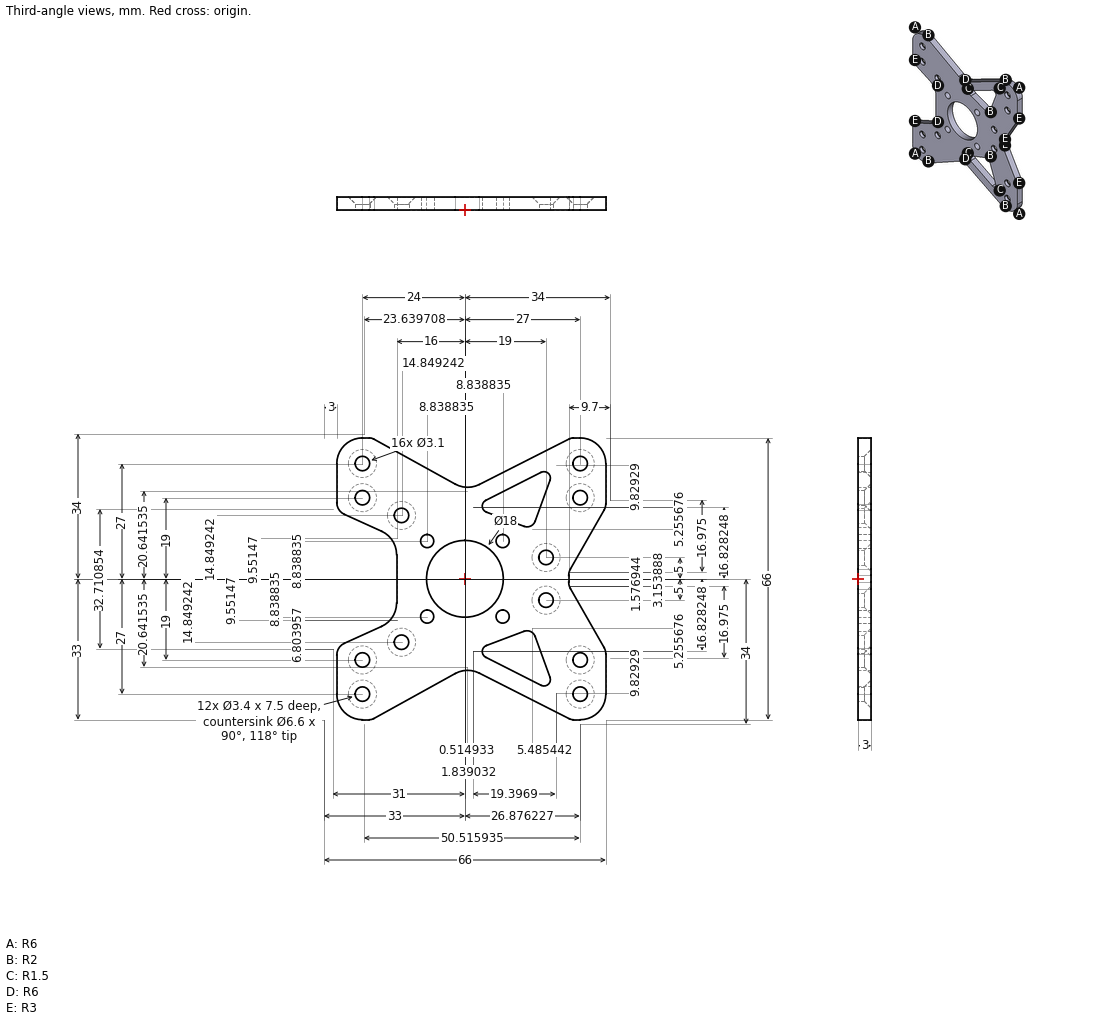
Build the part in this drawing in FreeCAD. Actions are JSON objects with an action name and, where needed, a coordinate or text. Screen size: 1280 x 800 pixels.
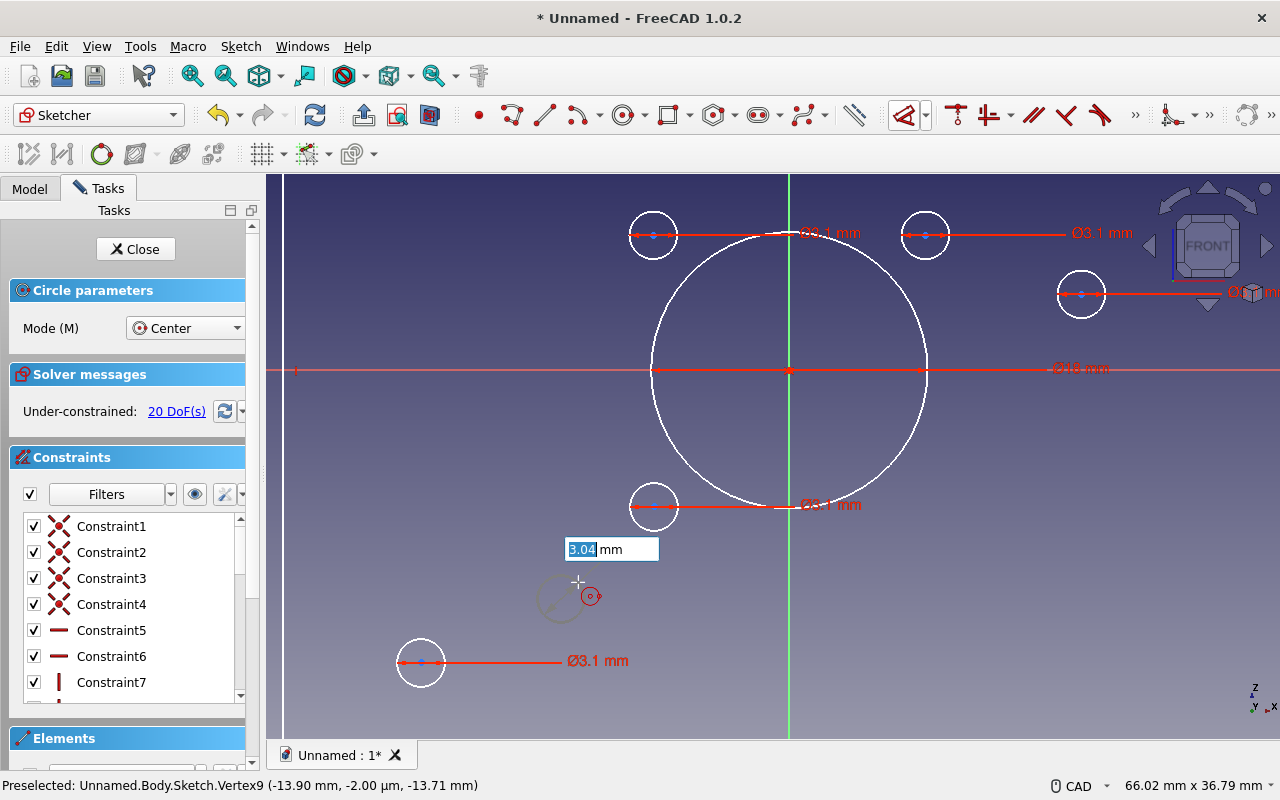
{"action": "type", "text": "3.1"}
{"action": "key", "text": "Return"}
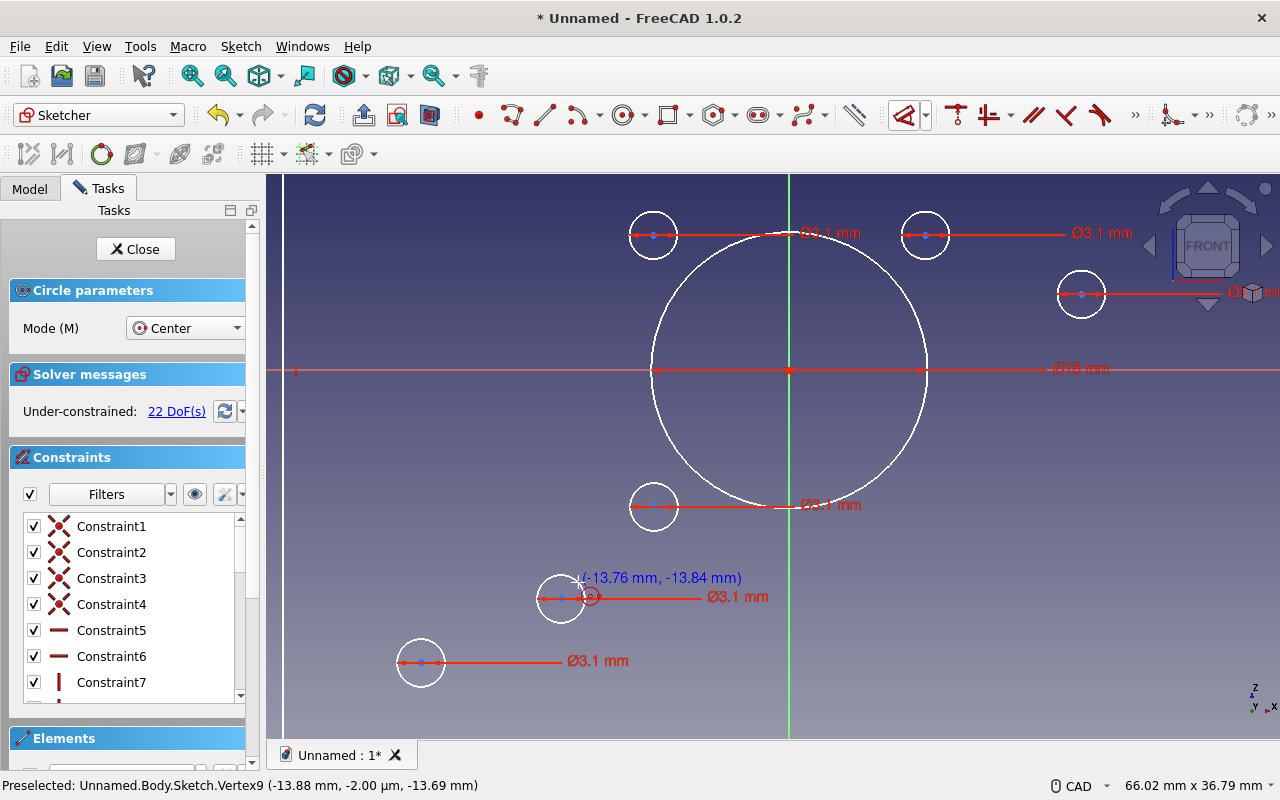
{"action": "scroll", "coordinate": [655, 507], "scroll_direction": "down", "scroll_amount": 5}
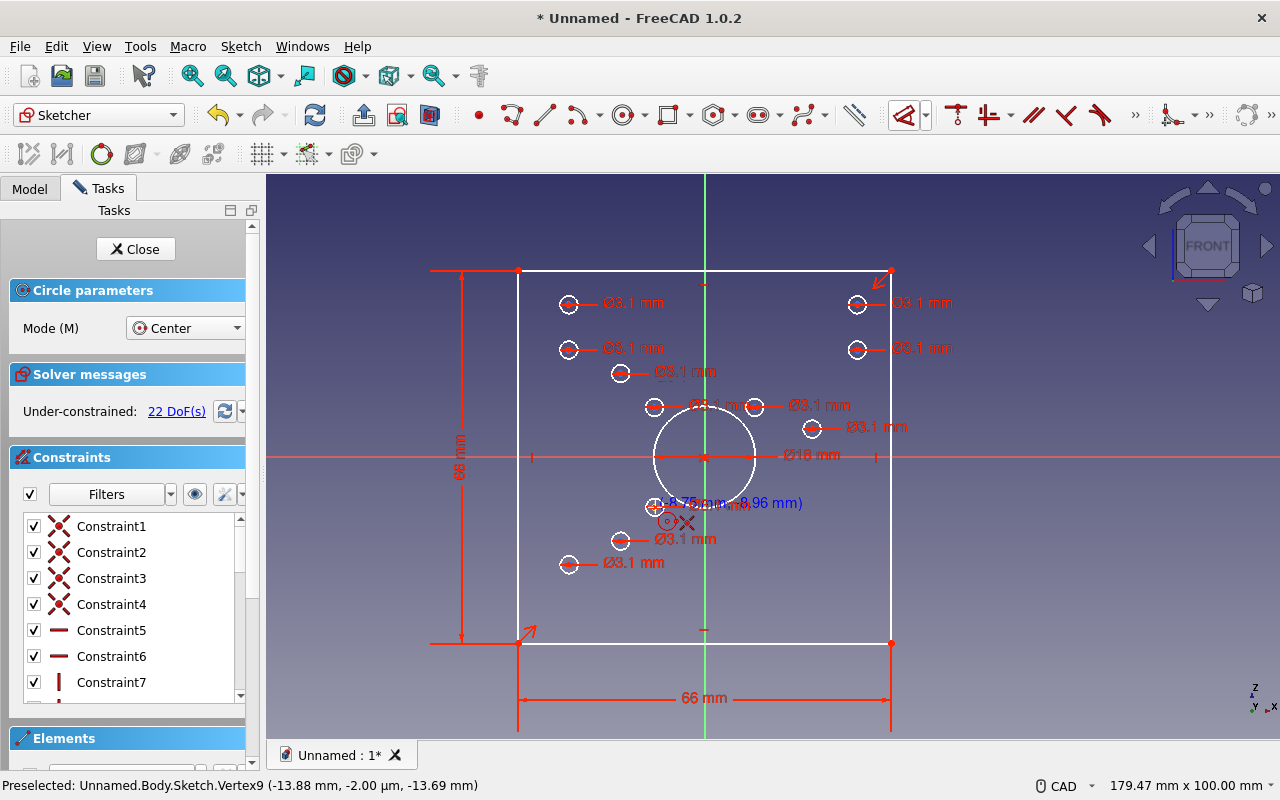
{"action": "scroll", "coordinate": [569, 610], "scroll_direction": "up", "scroll_amount": 5}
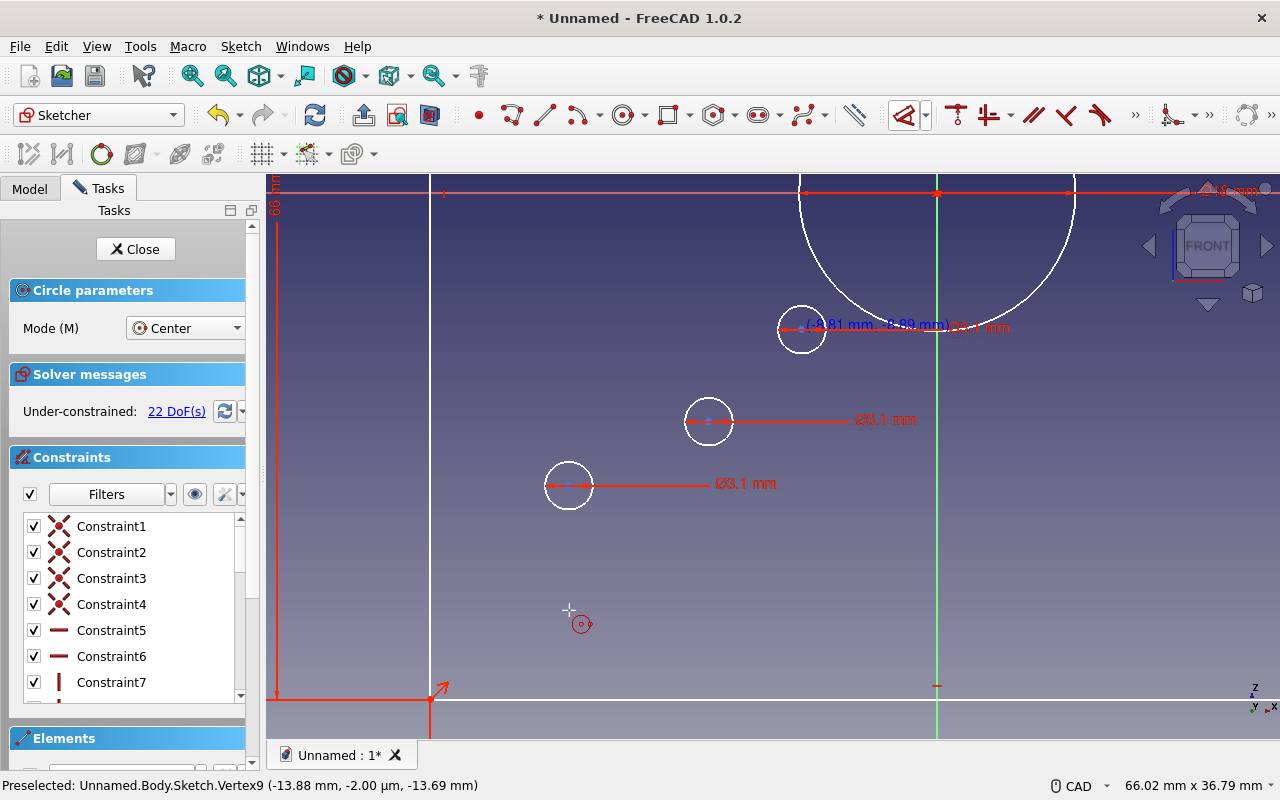
{"action": "left_click", "coordinate": [569, 608]}
{"action": "mouse_move", "coordinate": [585, 591]}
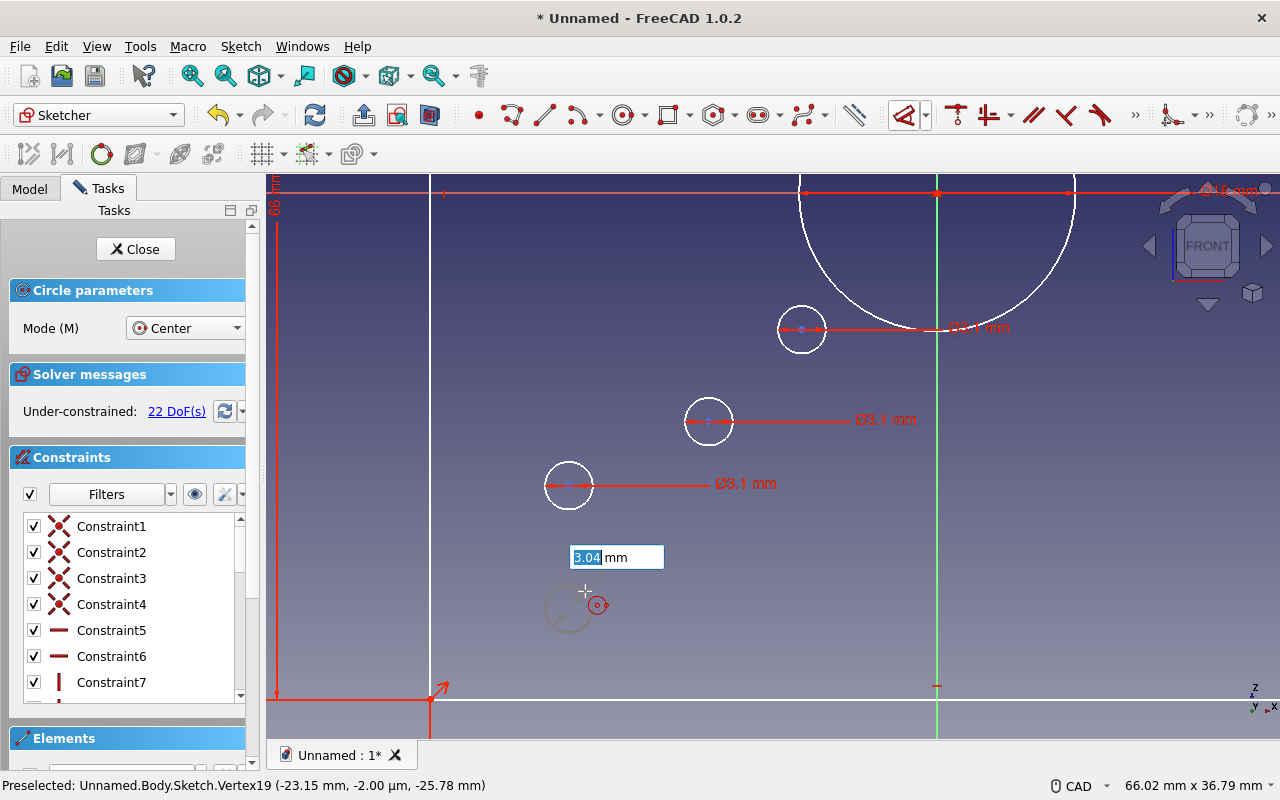
{"action": "type", "text": "3.1"}
{"action": "key", "text": "Return"}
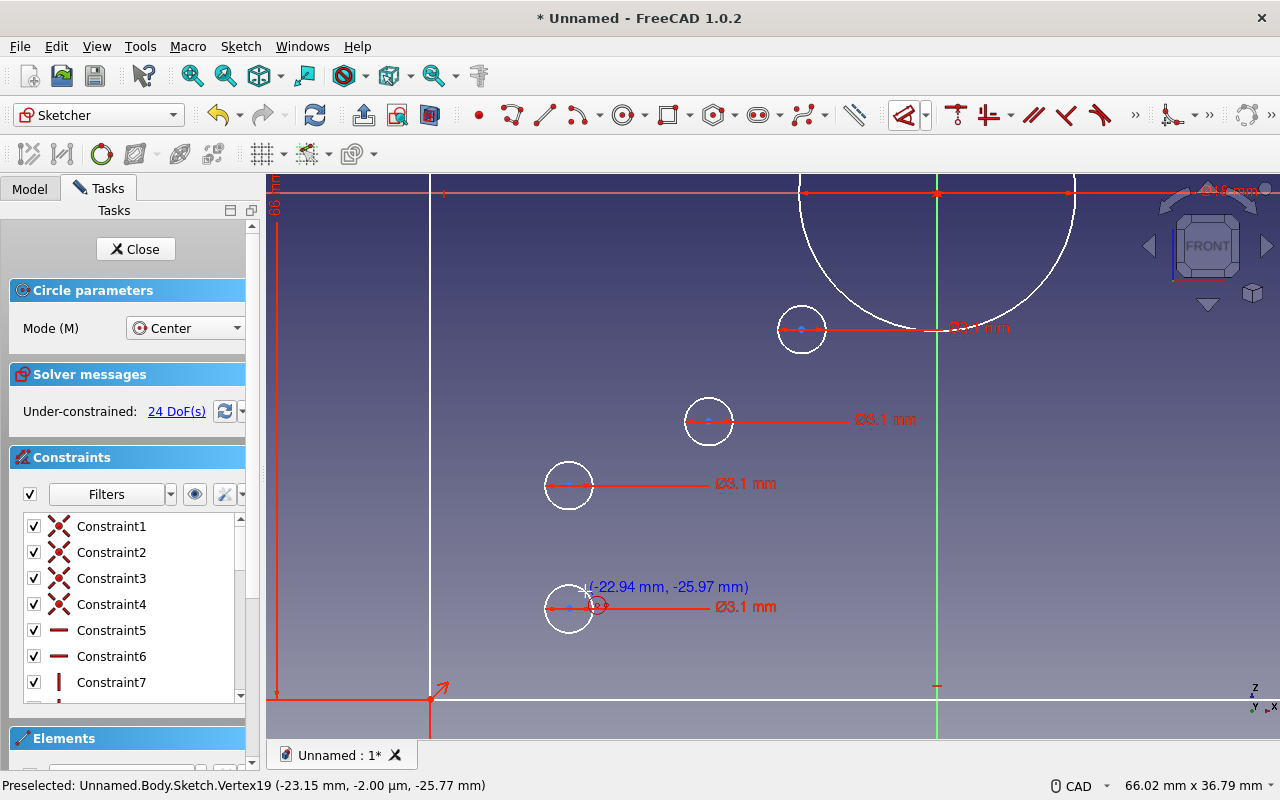
{"action": "left_click", "coordinate": [1073, 329]}
{"action": "mouse_move", "coordinate": [1090, 312]}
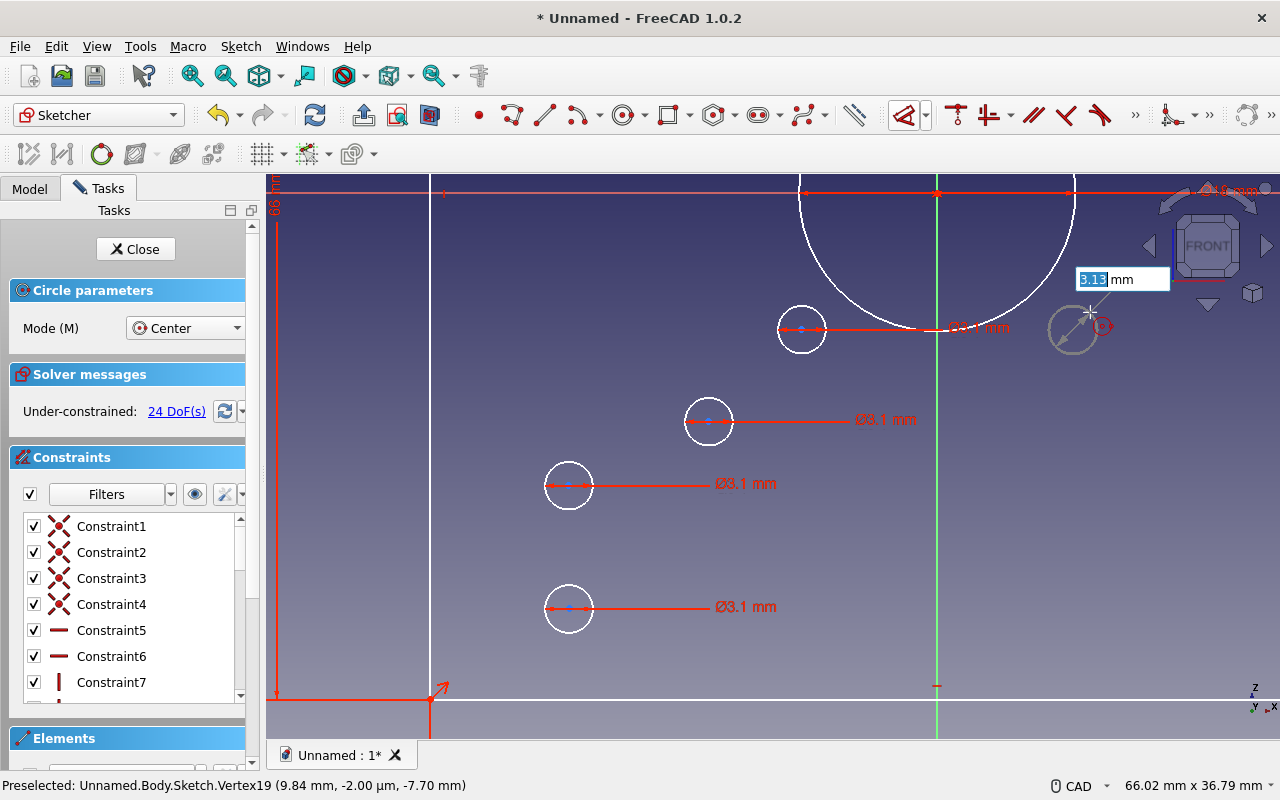
{"action": "type", "text": "3.1"}
{"action": "key", "text": "Return"}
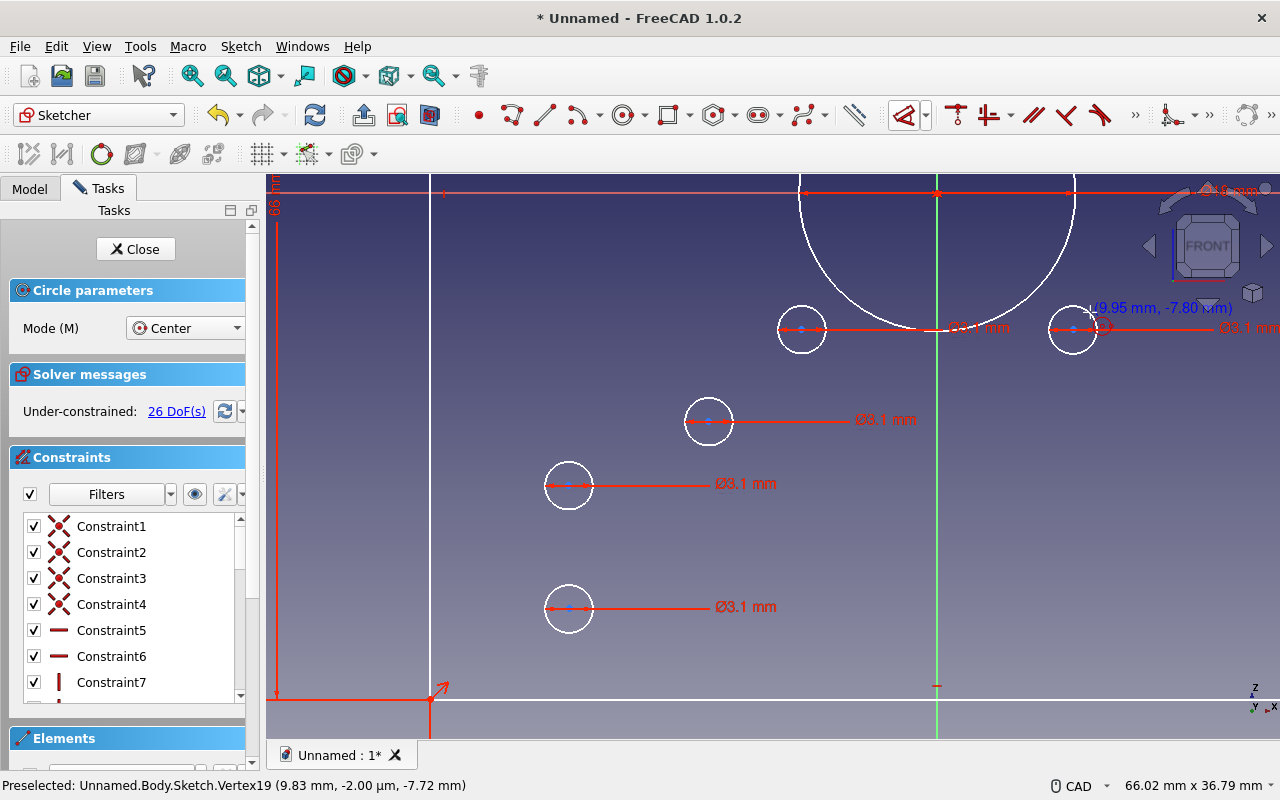
{"action": "scroll", "coordinate": [569, 610], "scroll_direction": "down", "scroll_amount": 5}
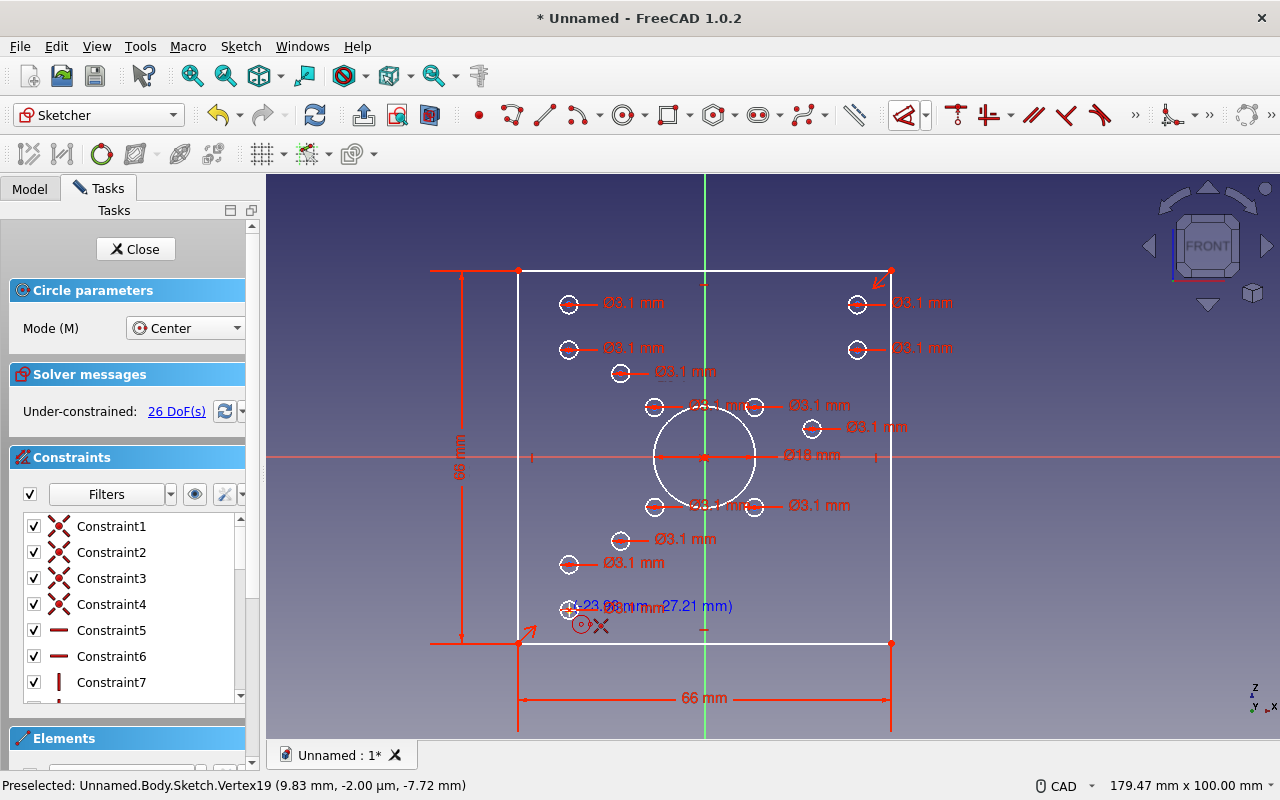
{"action": "scroll", "coordinate": [812, 485], "scroll_direction": "up", "scroll_amount": 5}